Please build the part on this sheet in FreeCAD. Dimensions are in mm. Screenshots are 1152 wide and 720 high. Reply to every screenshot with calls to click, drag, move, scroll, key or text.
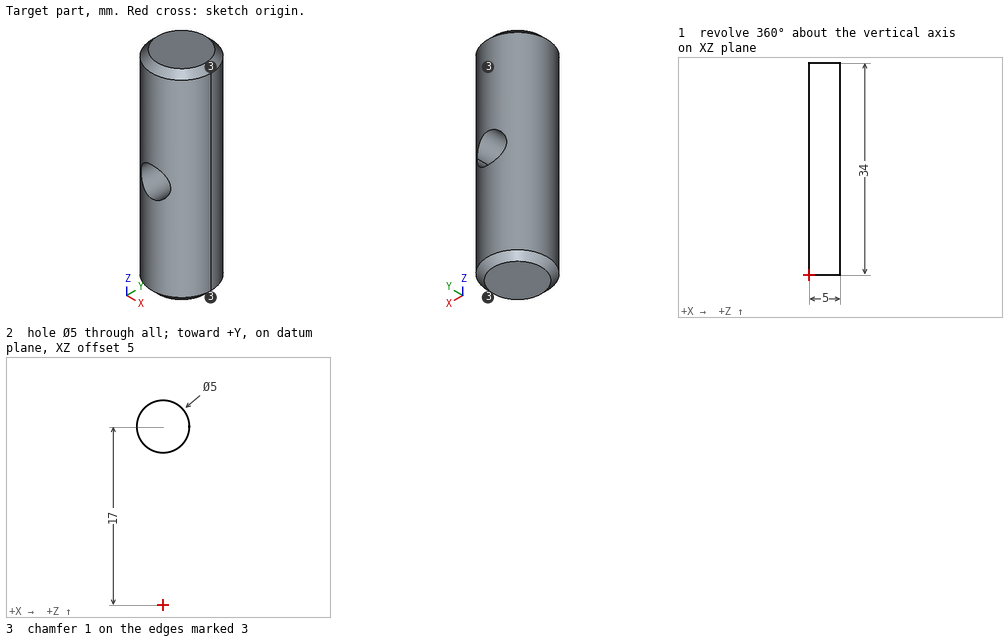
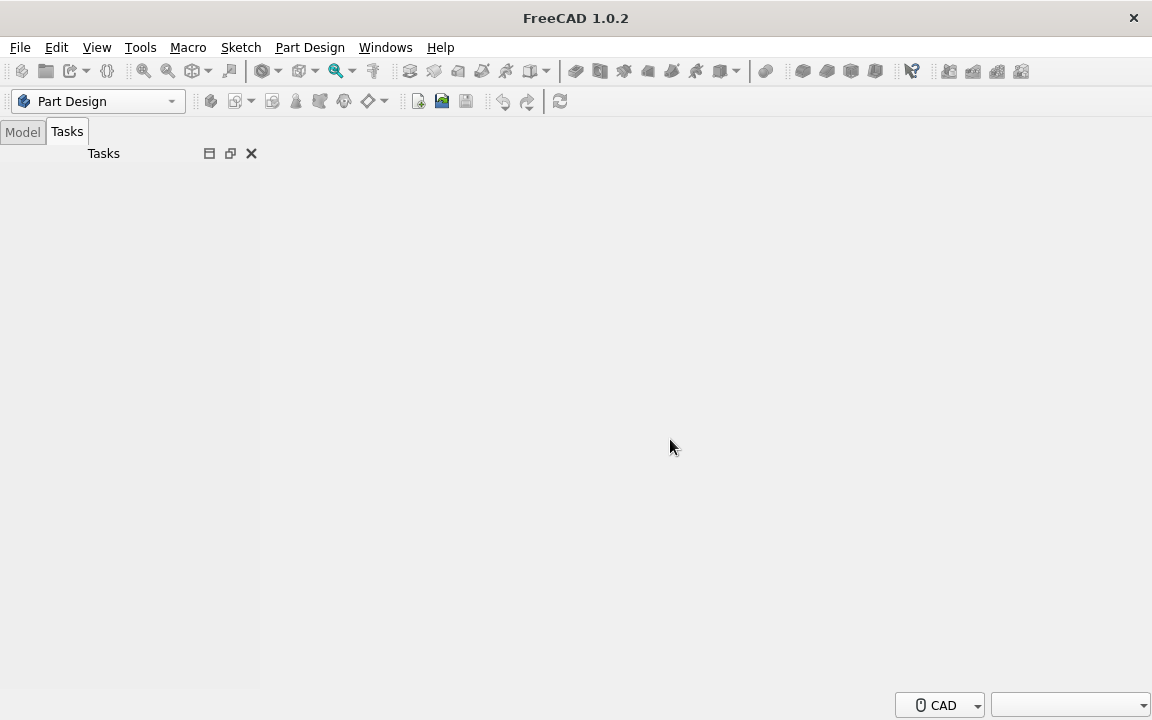
click(418, 102)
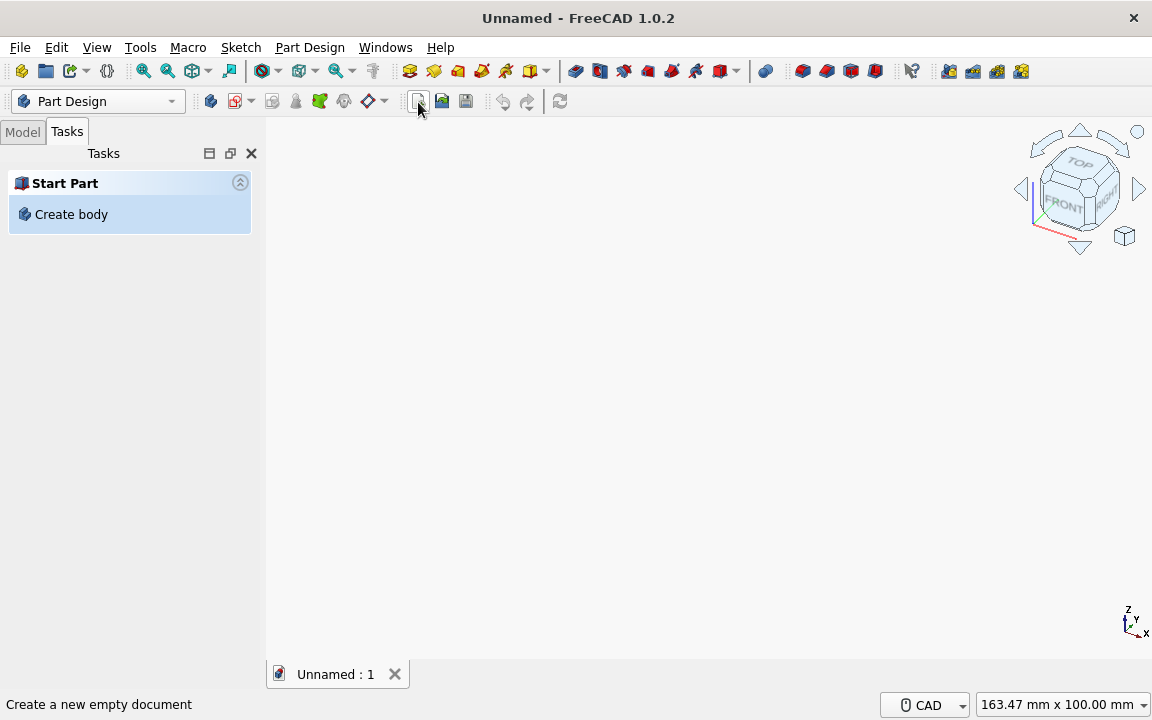
click(236, 102)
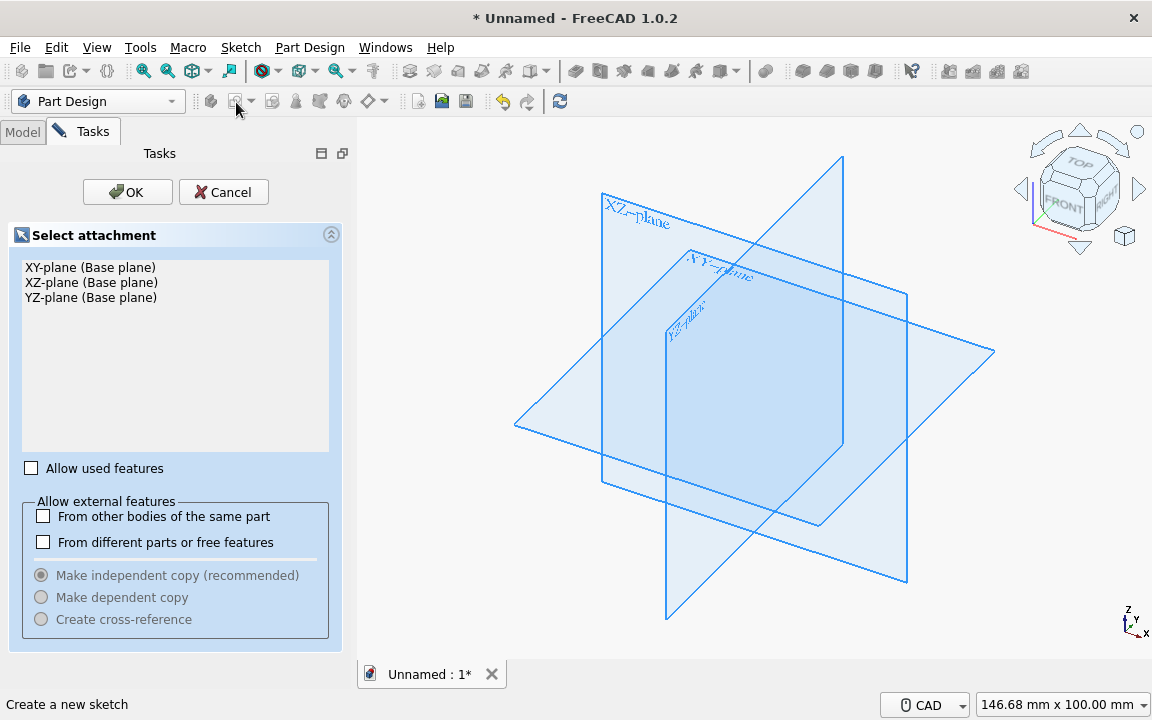
click(82, 282)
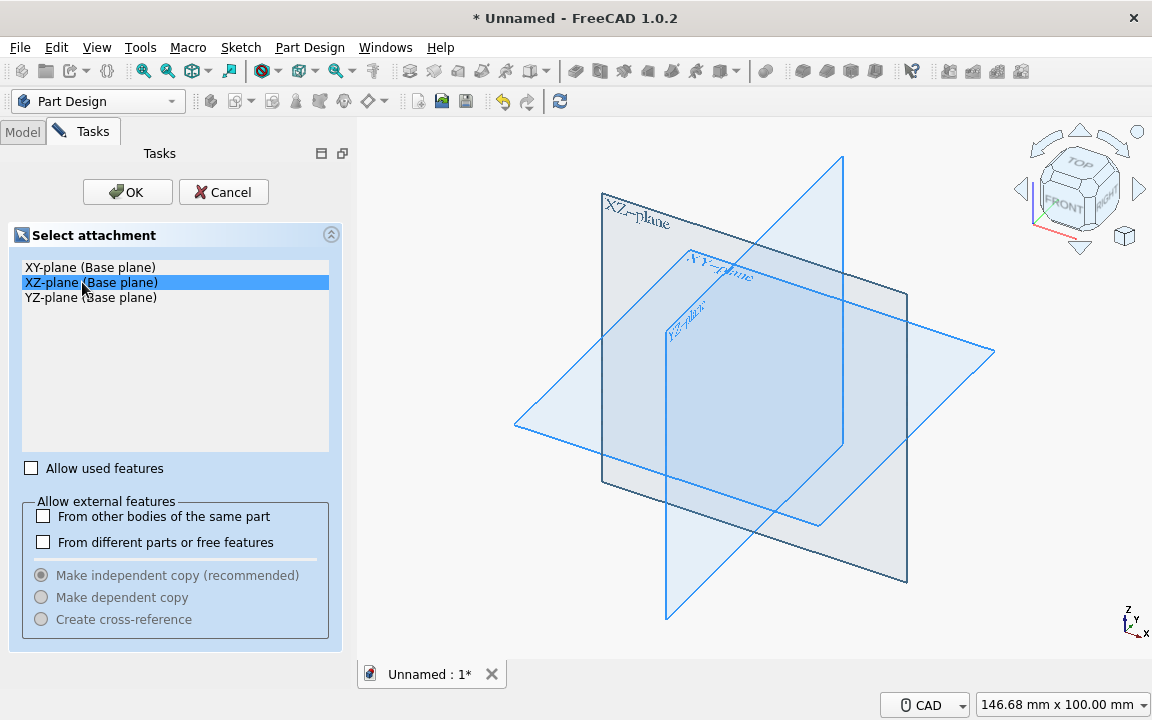
click(128, 192)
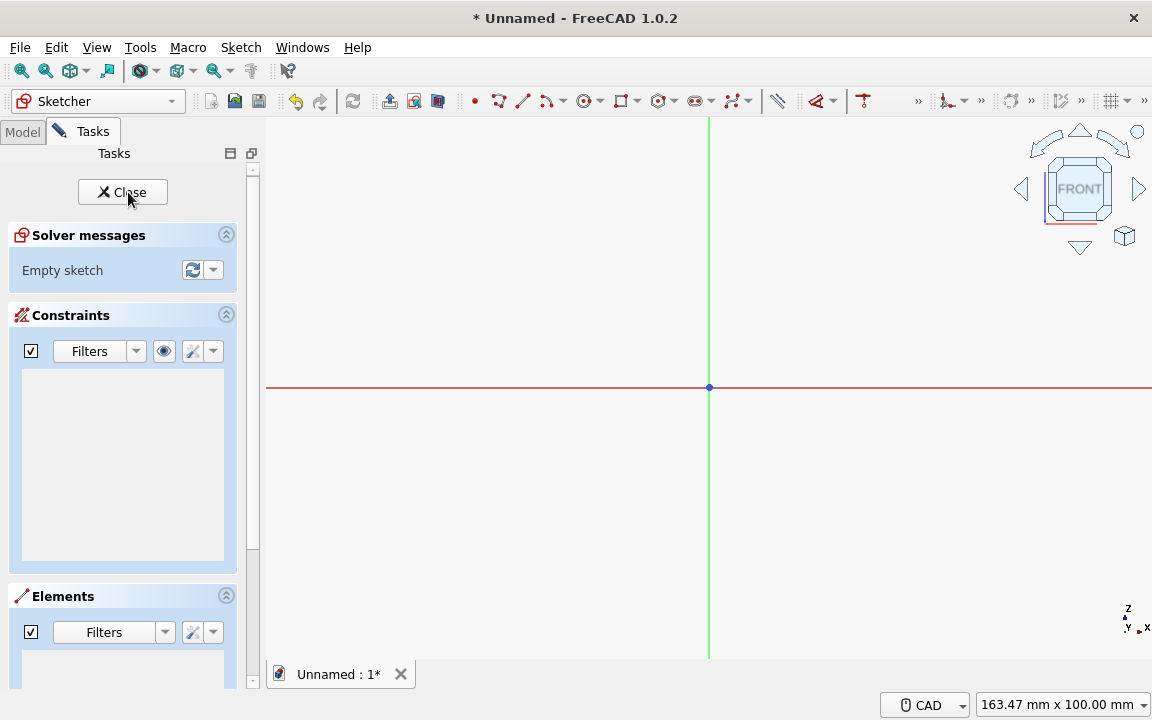
scroll(822, 184, up, 3)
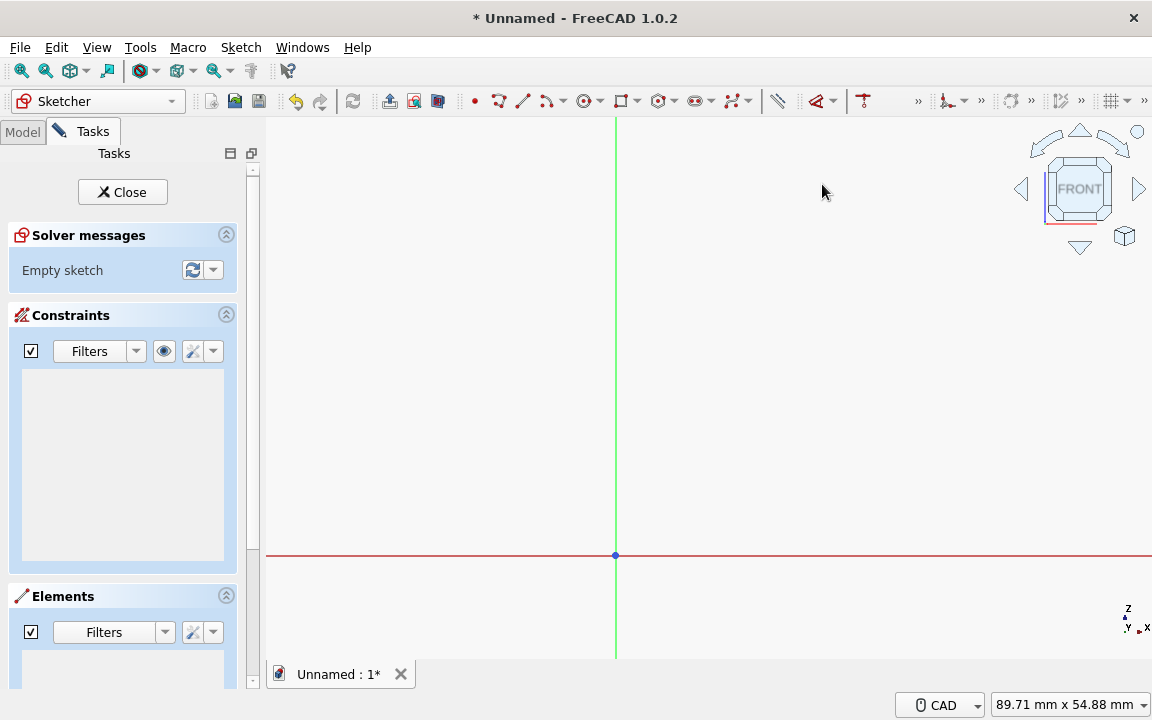
click(622, 102)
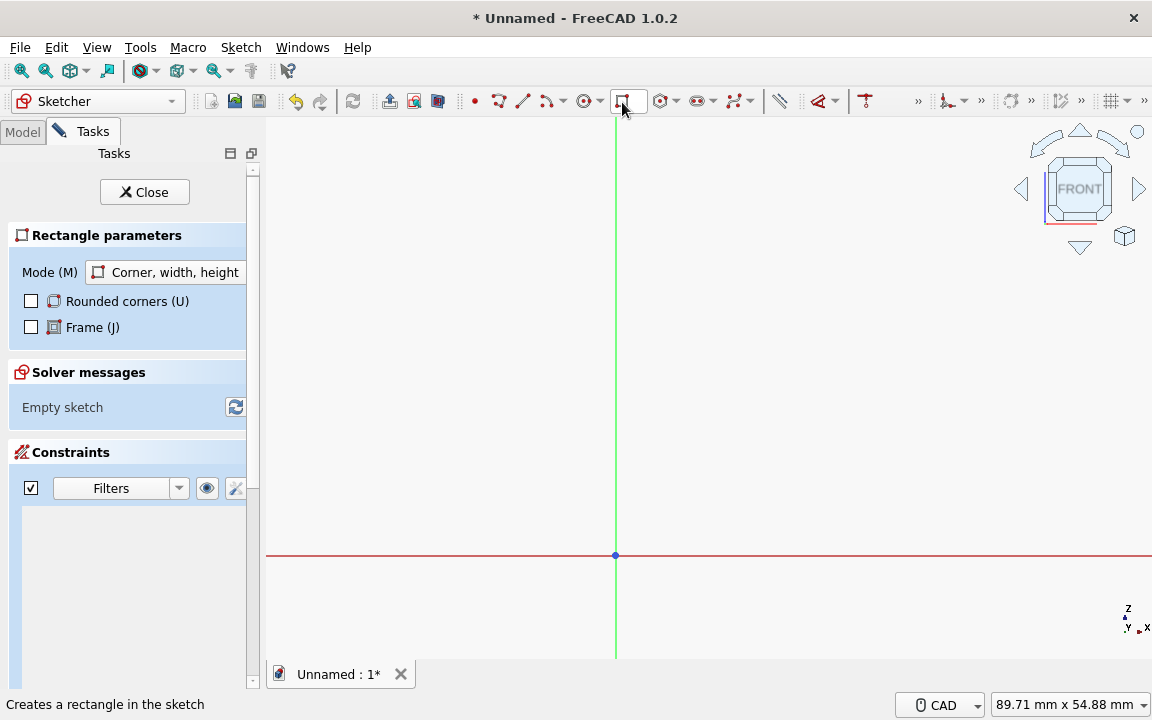
click(616, 556)
click(665, 220)
key(Escape)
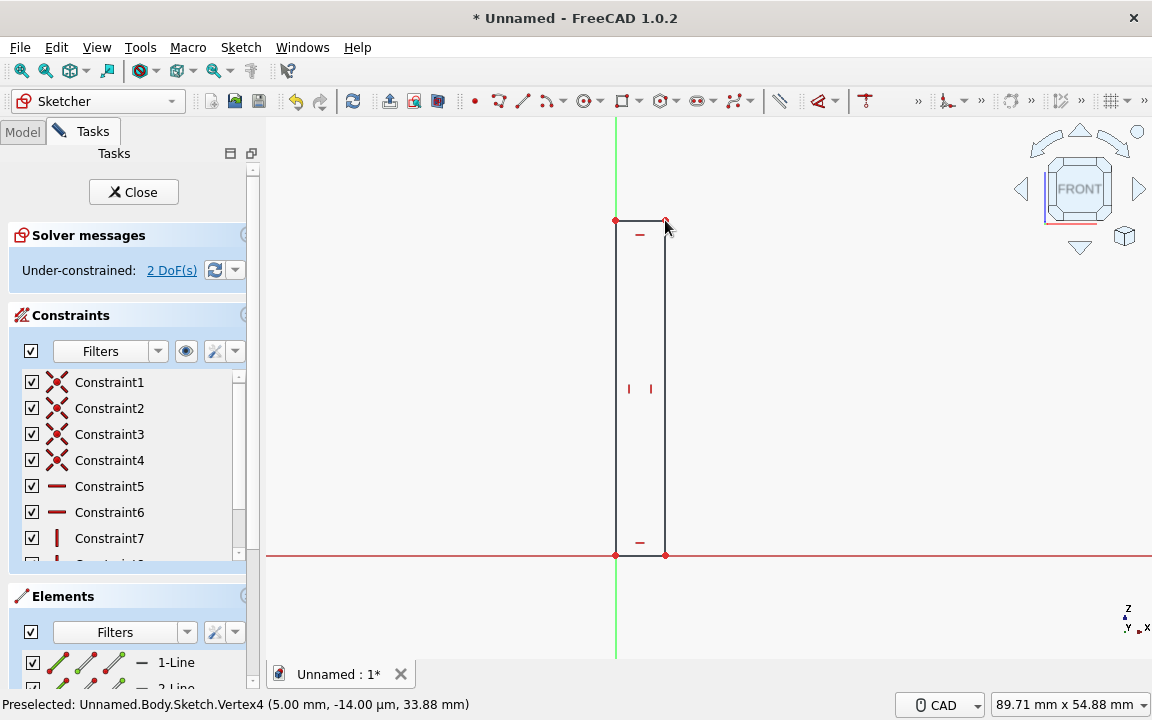
click(630, 556)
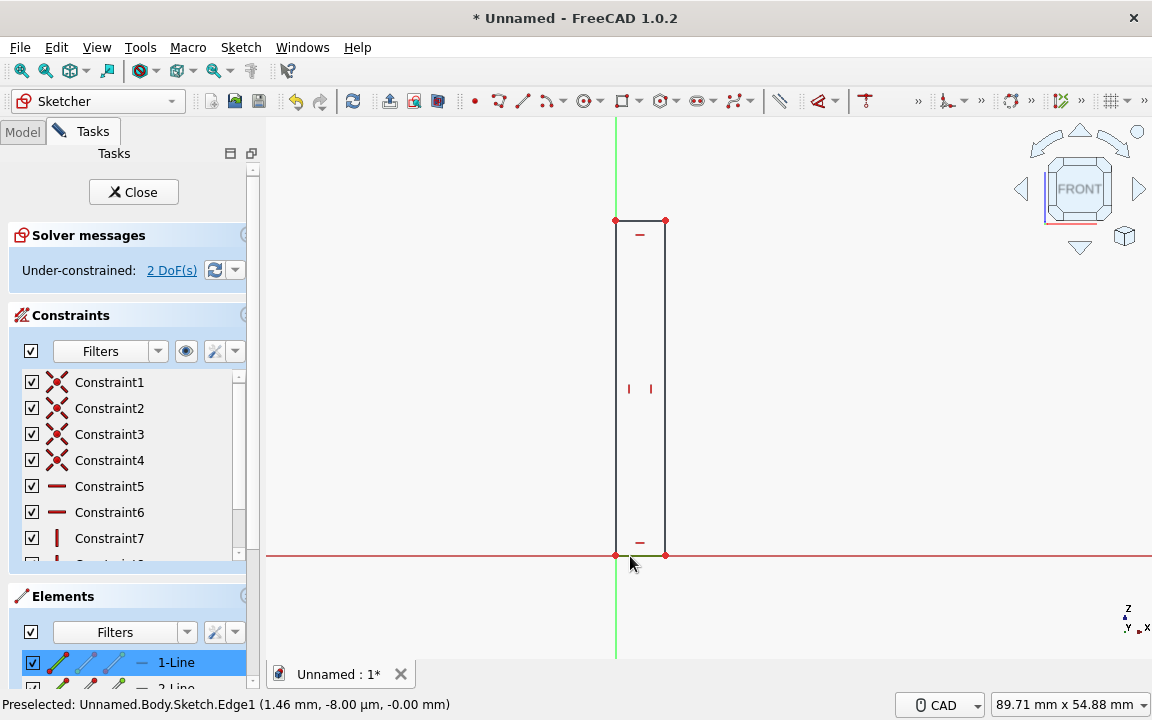
click(838, 102)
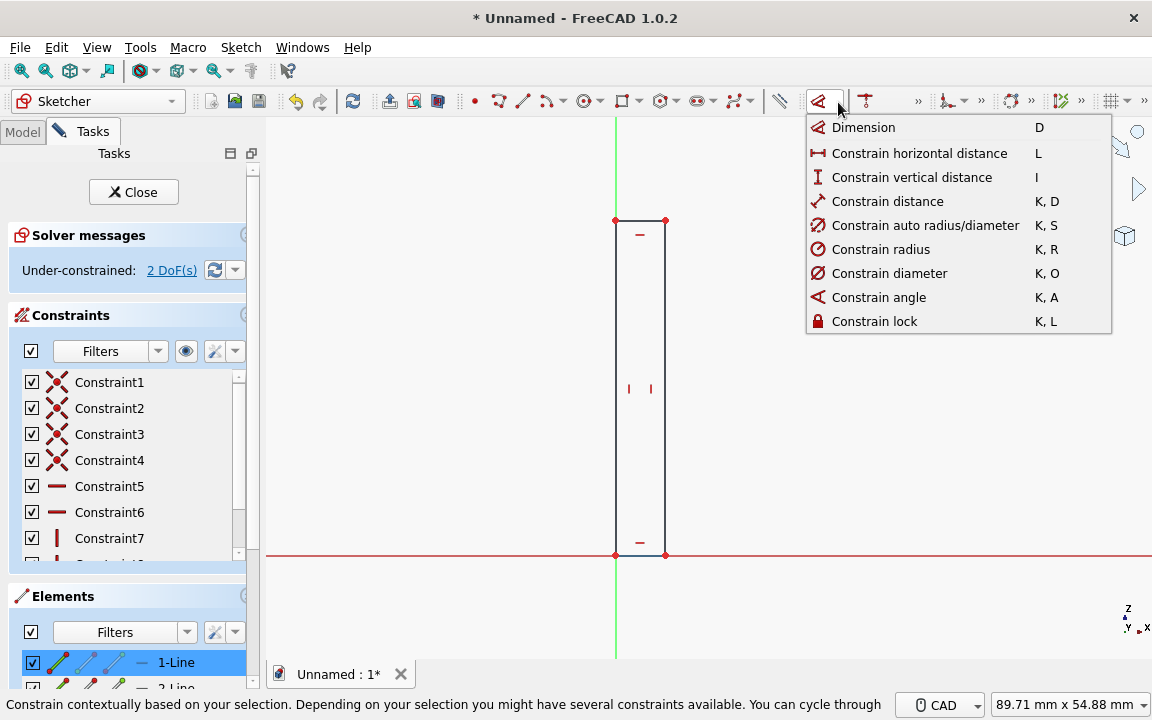
click(959, 153)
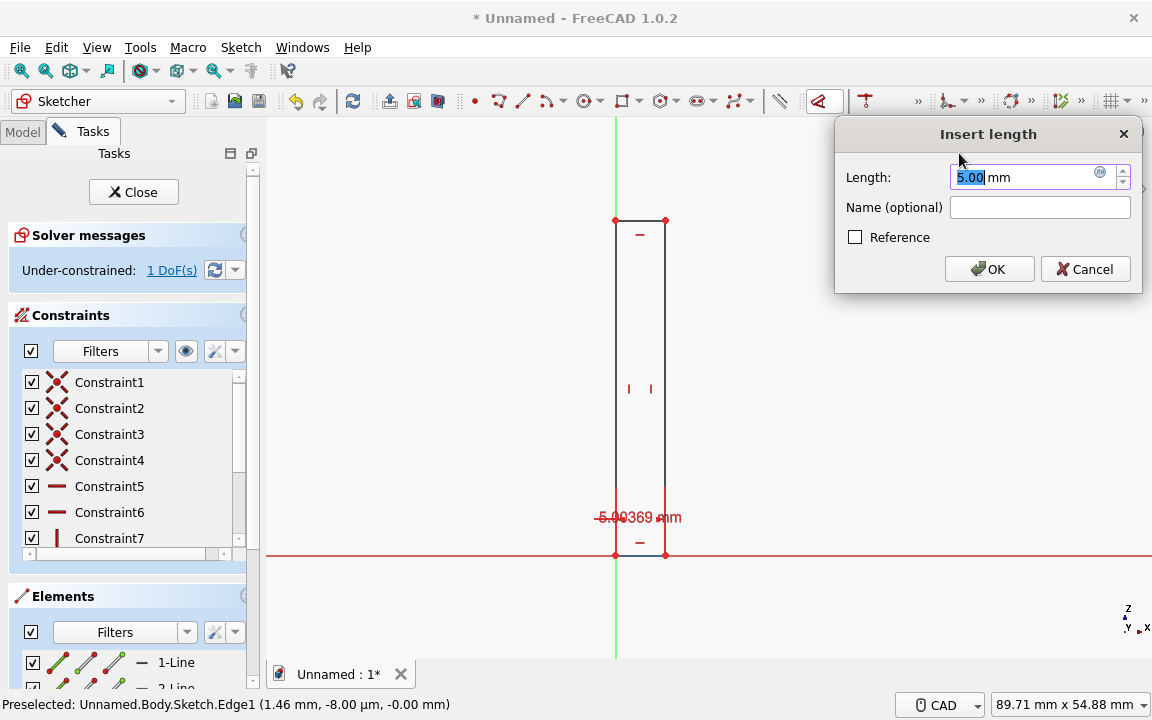
text(5)
key(Return)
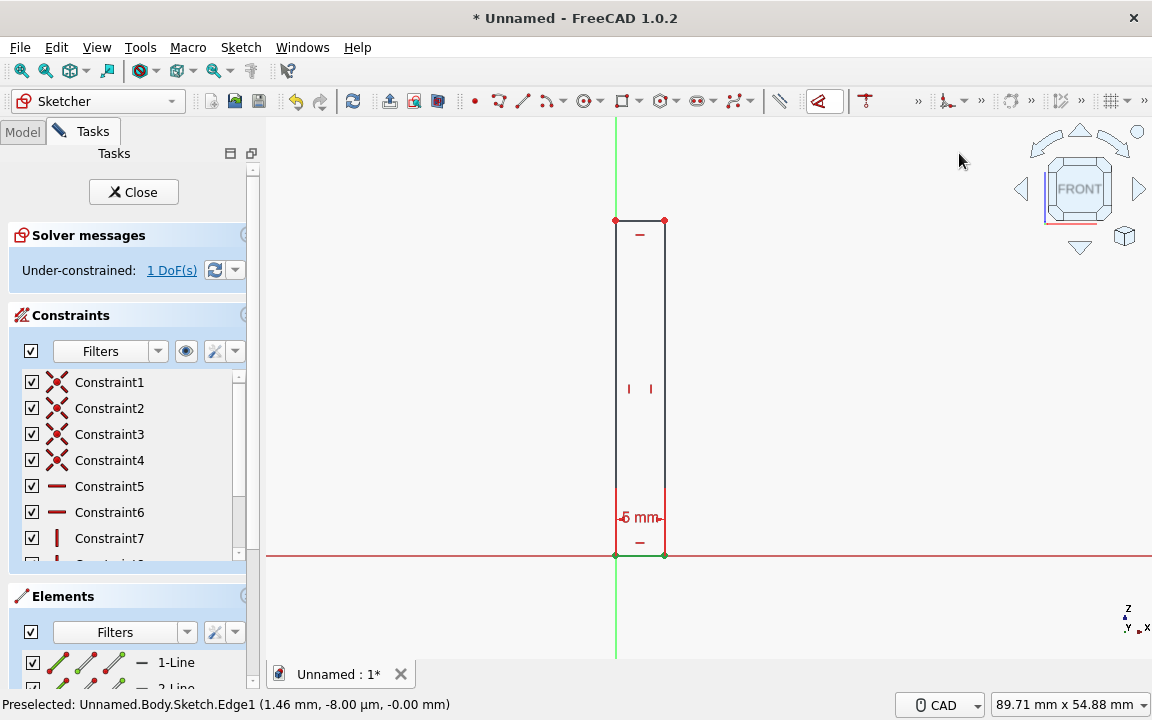
click(665, 455)